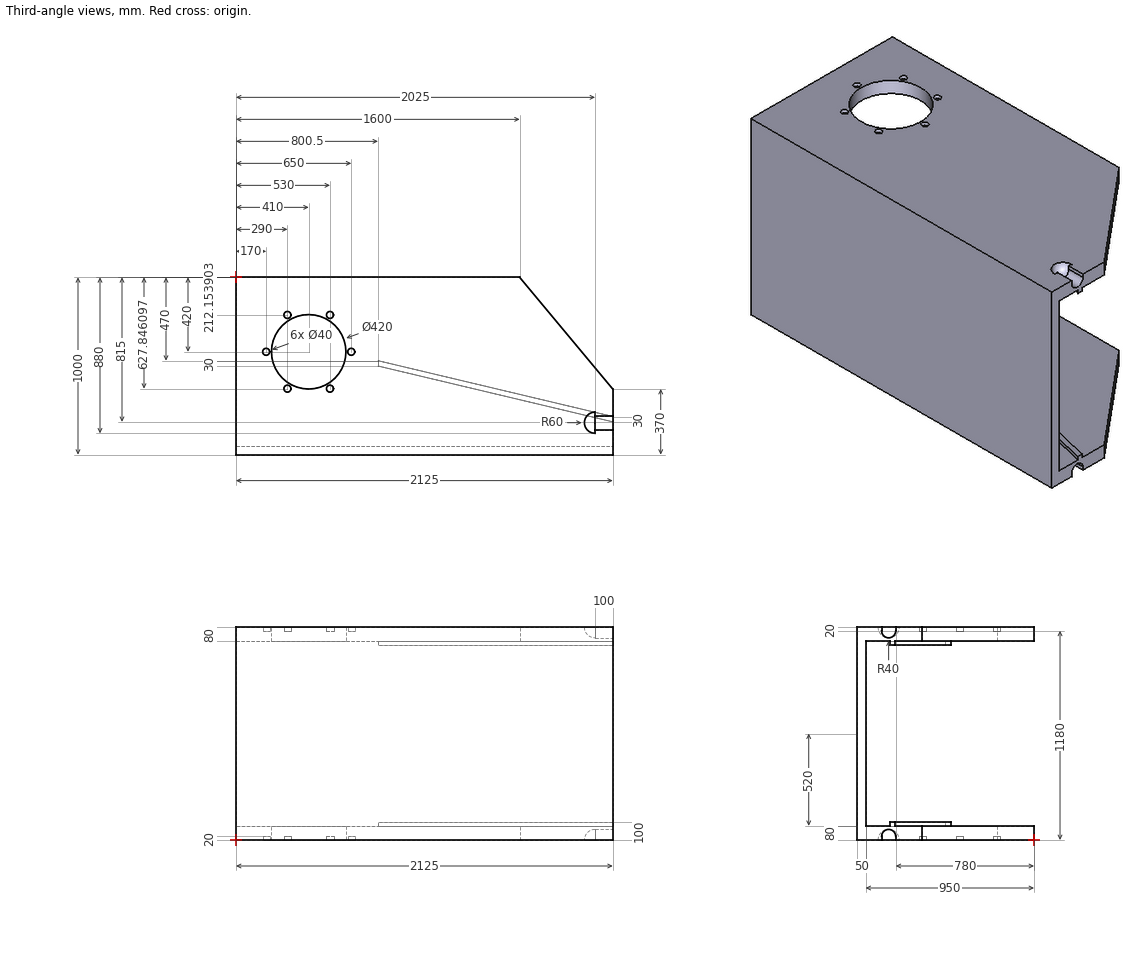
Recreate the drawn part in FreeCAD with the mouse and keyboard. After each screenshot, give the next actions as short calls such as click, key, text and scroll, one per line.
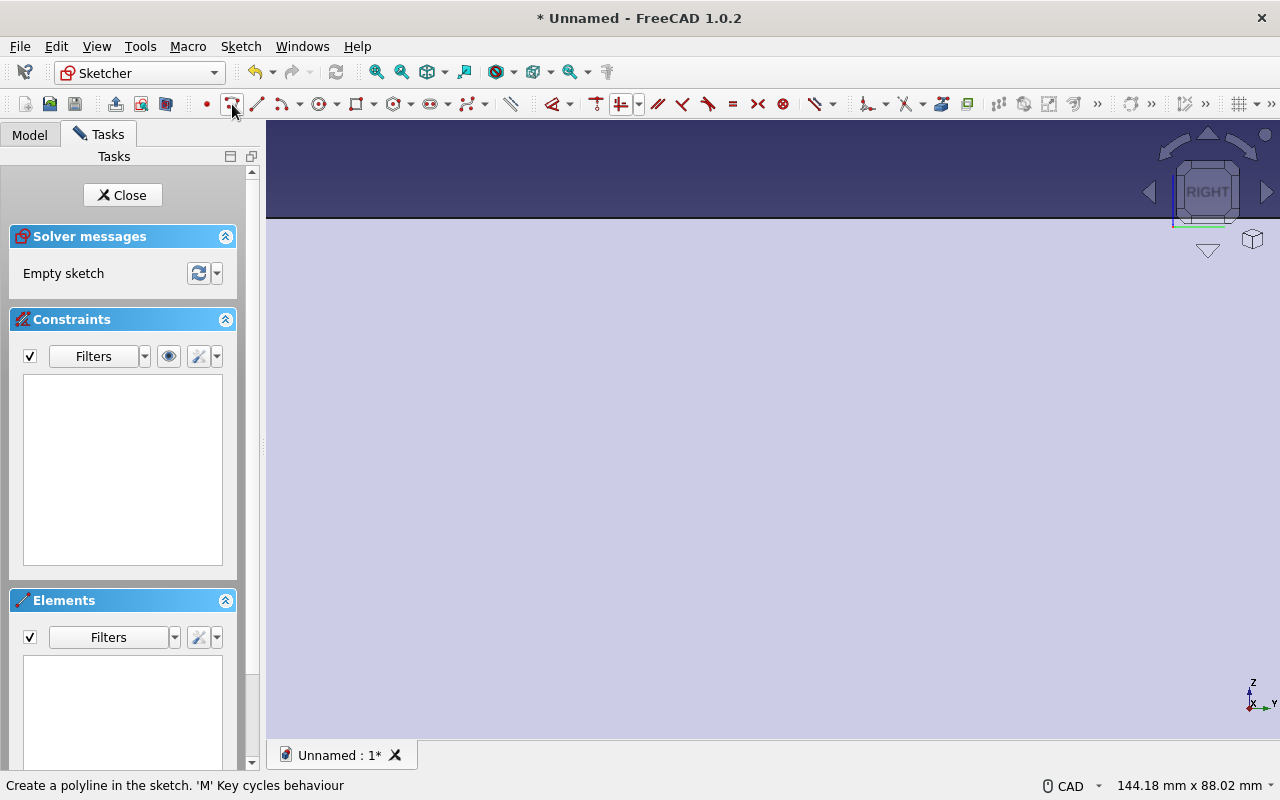
click(985, 359)
click(985, 218)
click(423, 218)
click(423, 359)
right_click(423, 359)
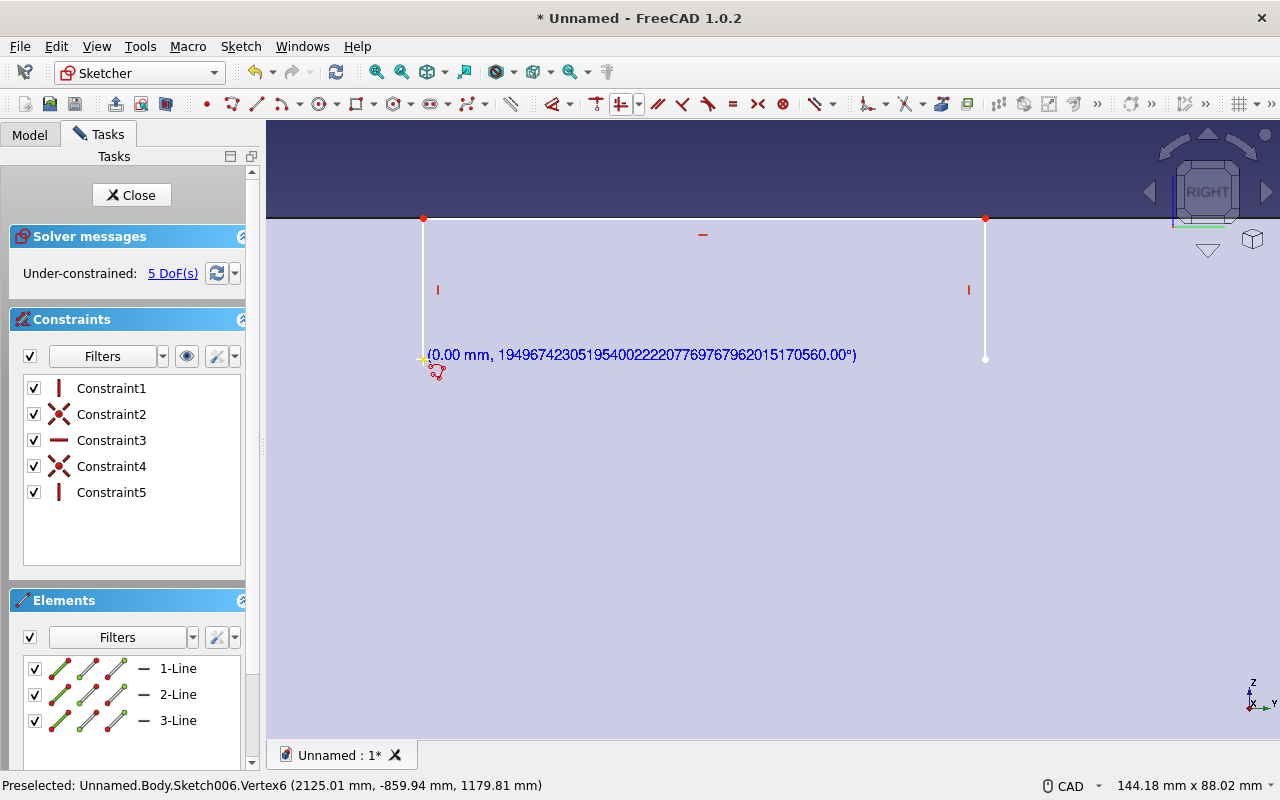
key(g)
key(3)
key(a)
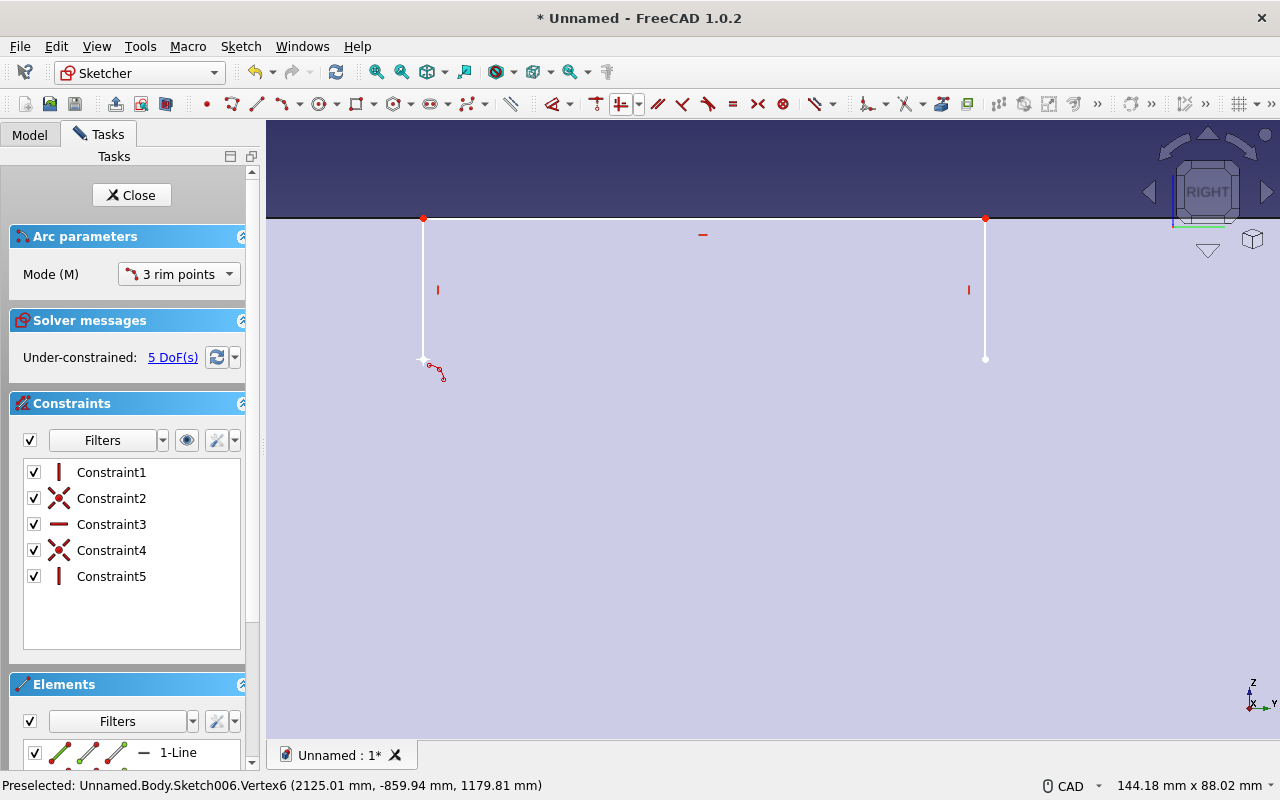
click(423, 360)
click(985, 360)
click(704, 640)
key(Escape)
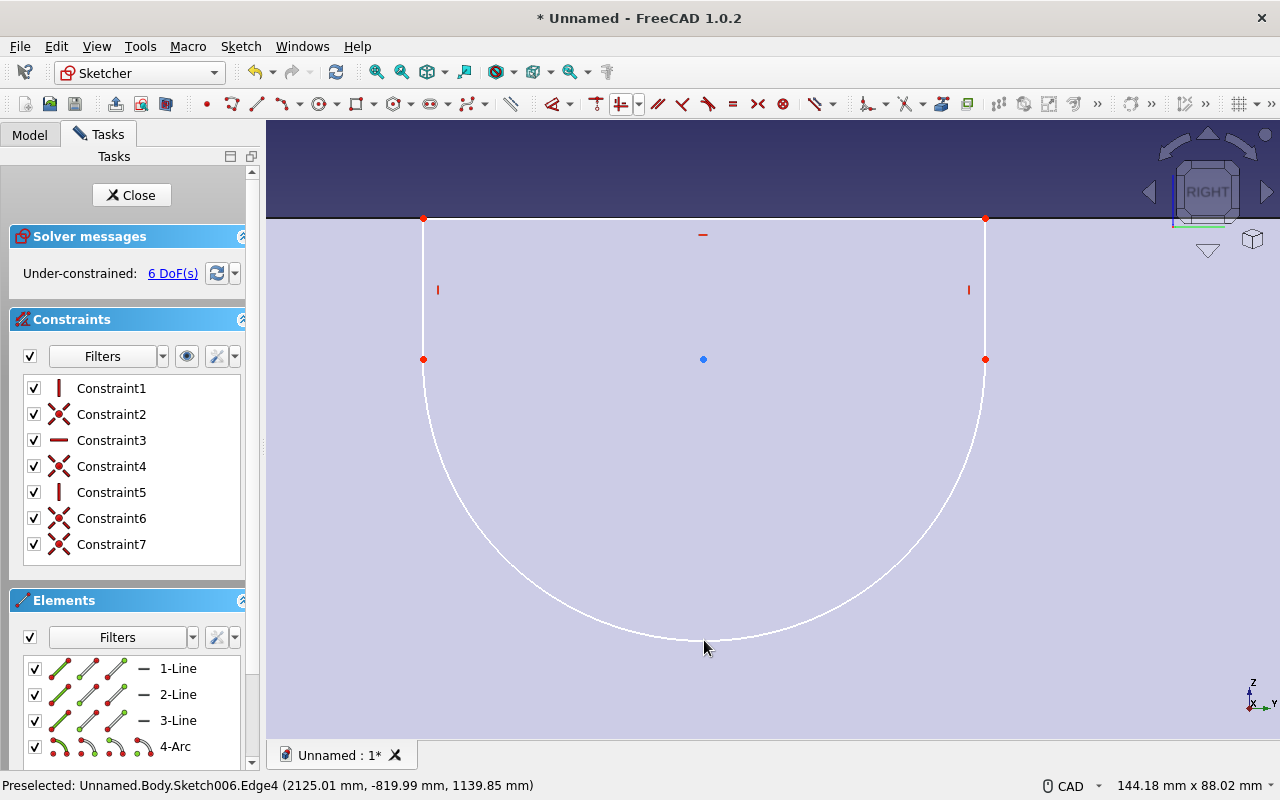
key(d)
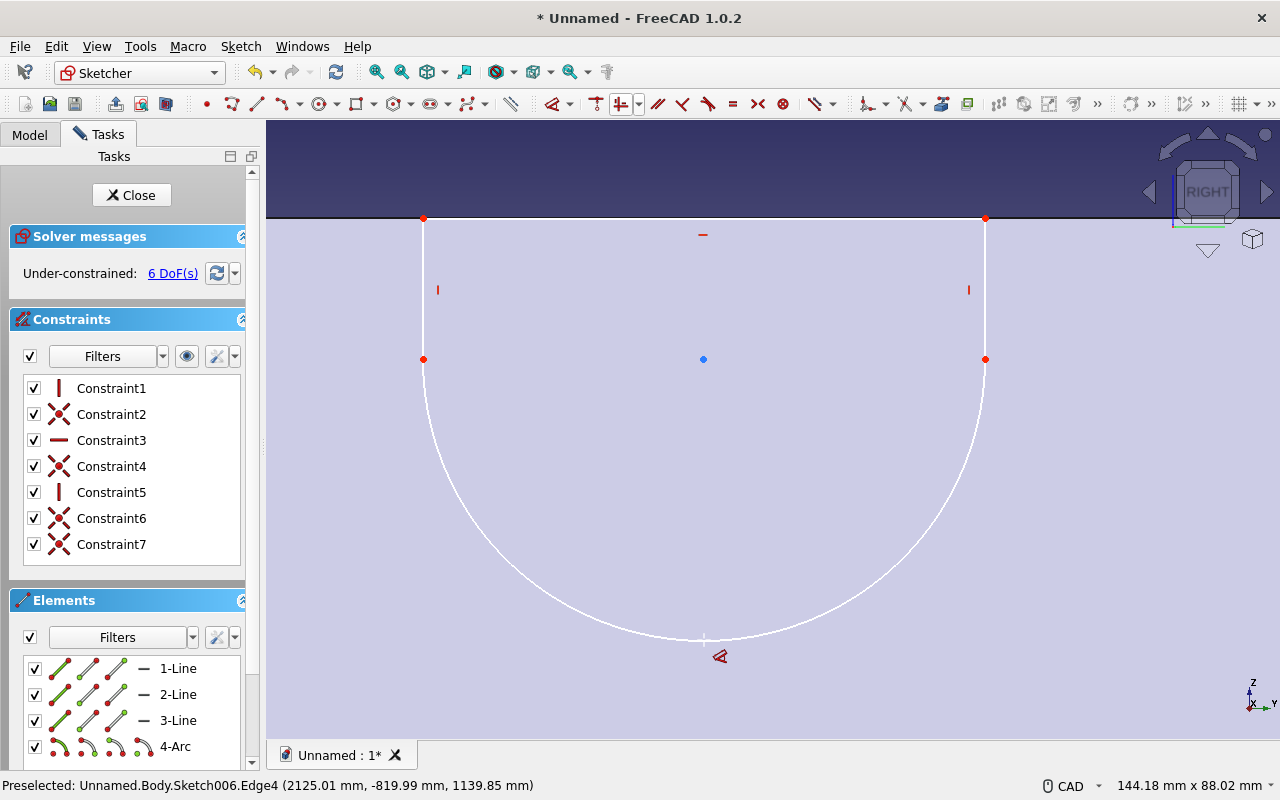
click(539, 587)
click(520, 613)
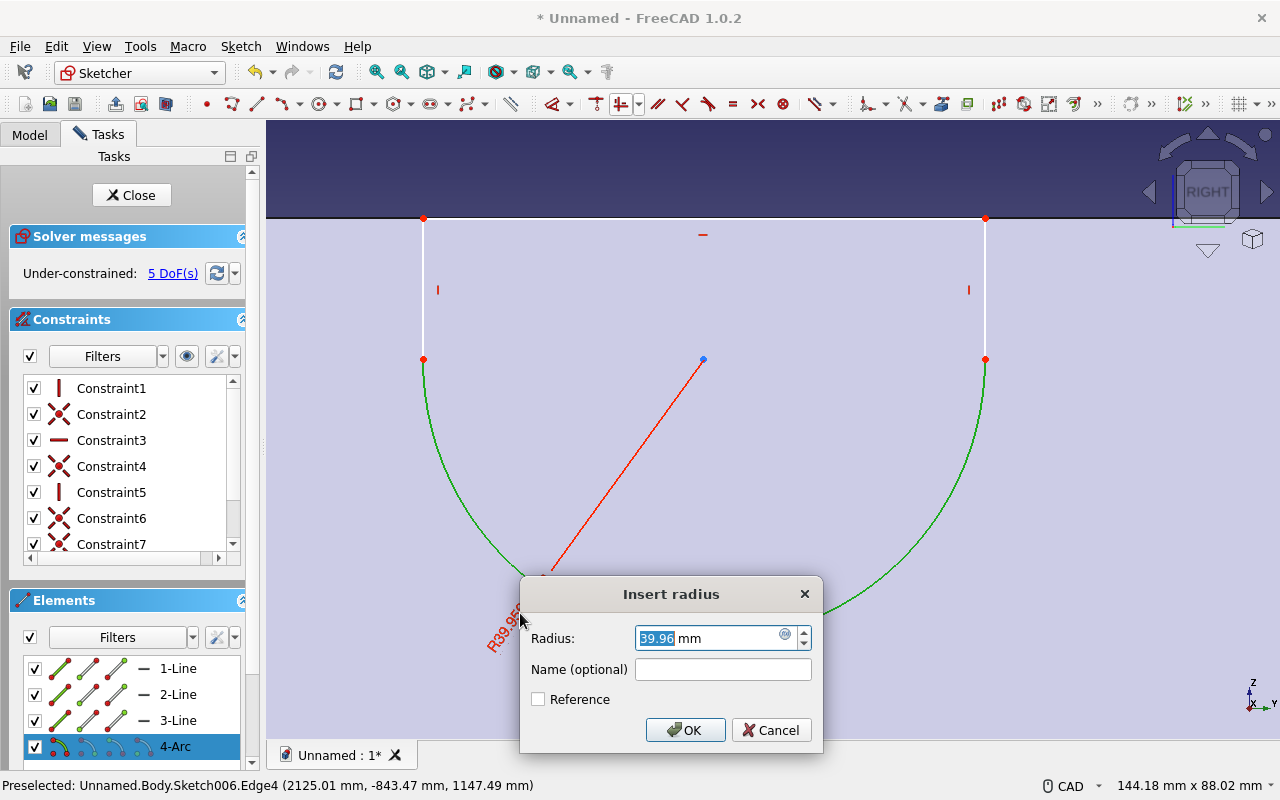
text(40)
key(Return)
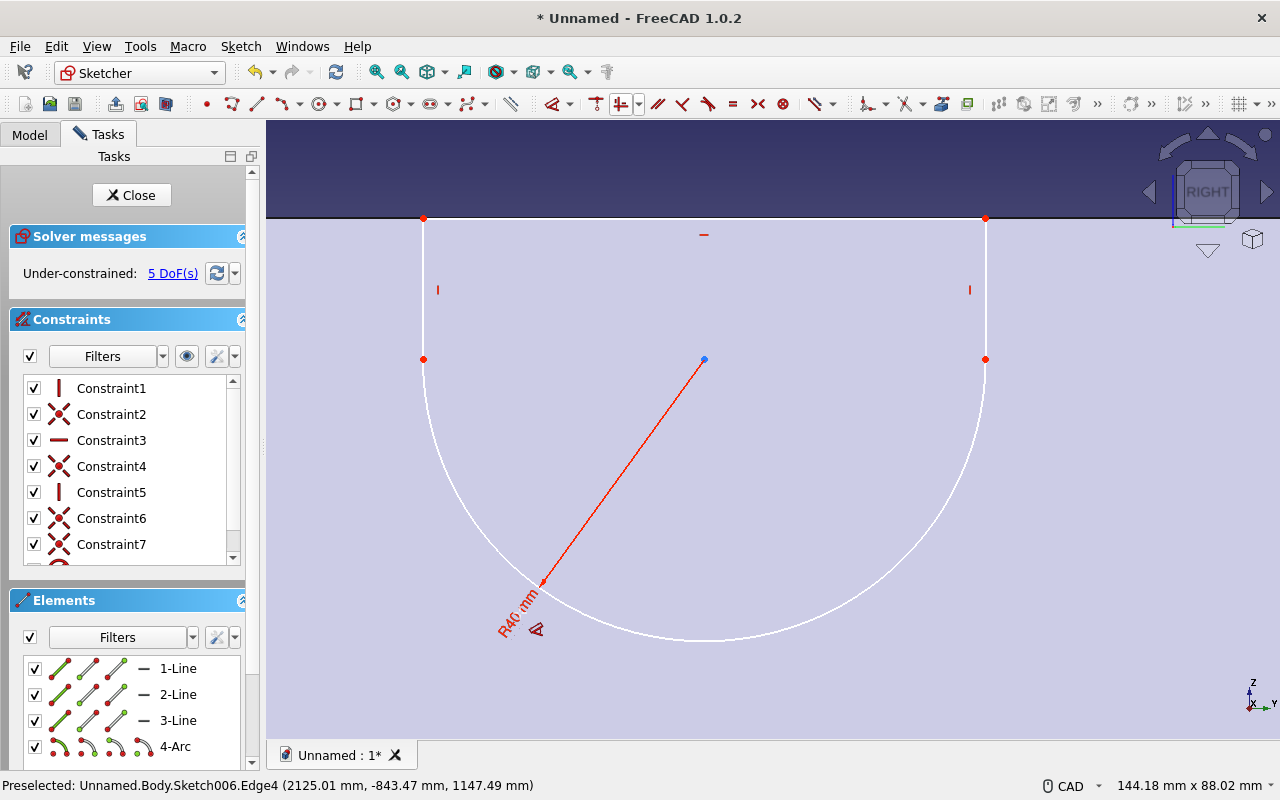
click(986, 318)
click(1020, 290)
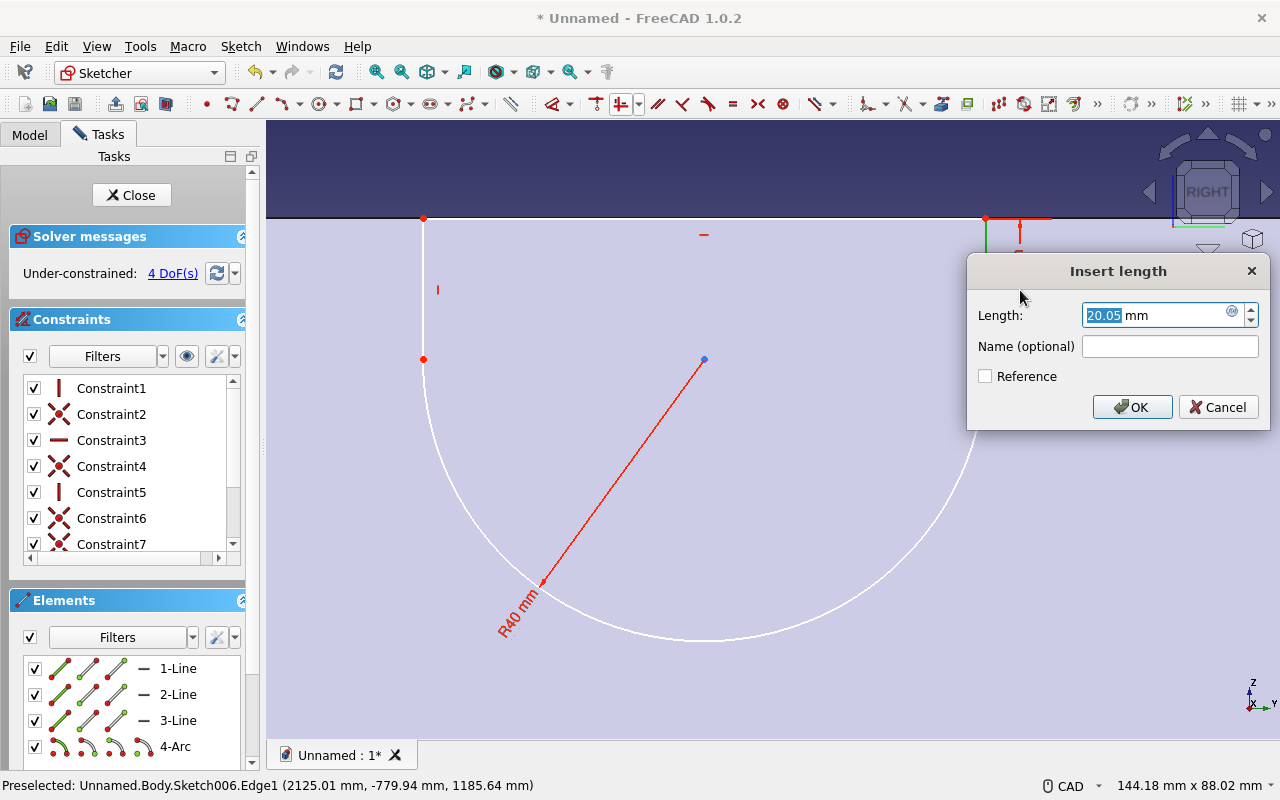
text(20)
key(Return)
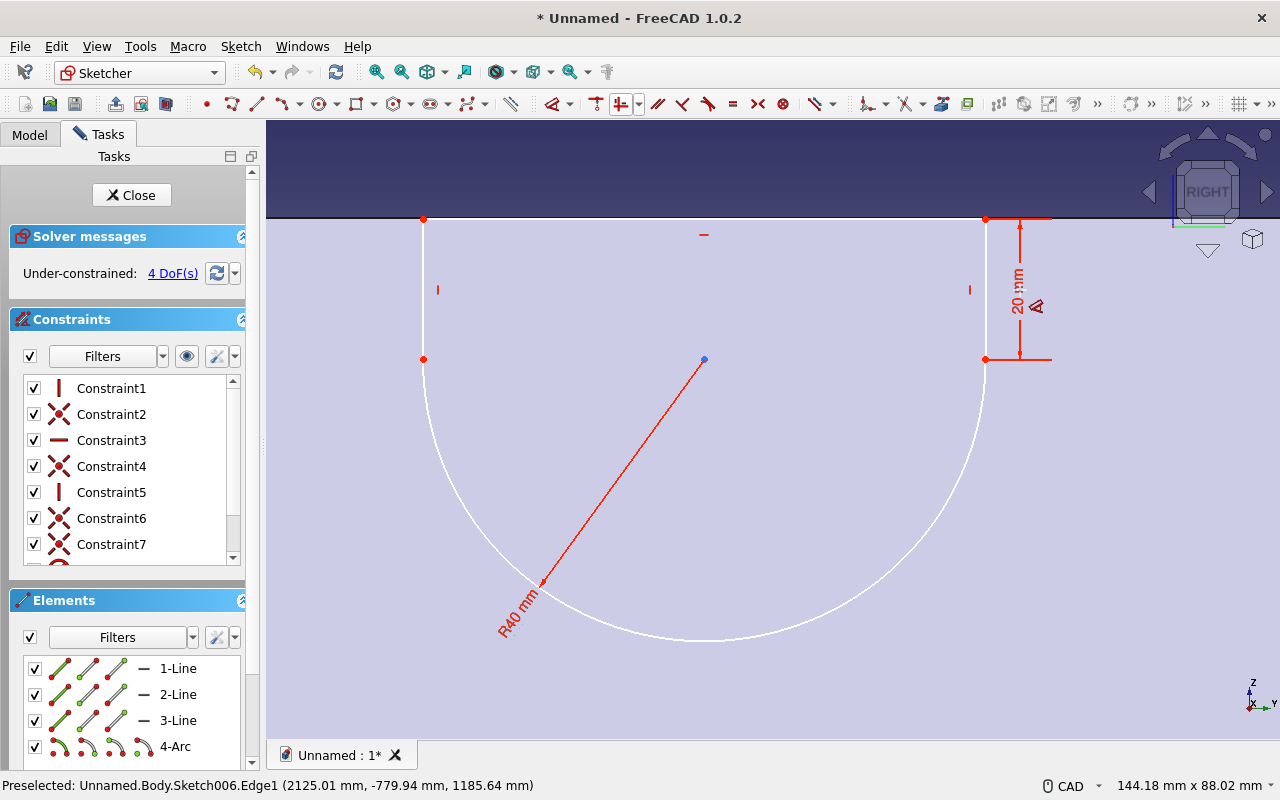
click(423, 262)
click(389, 290)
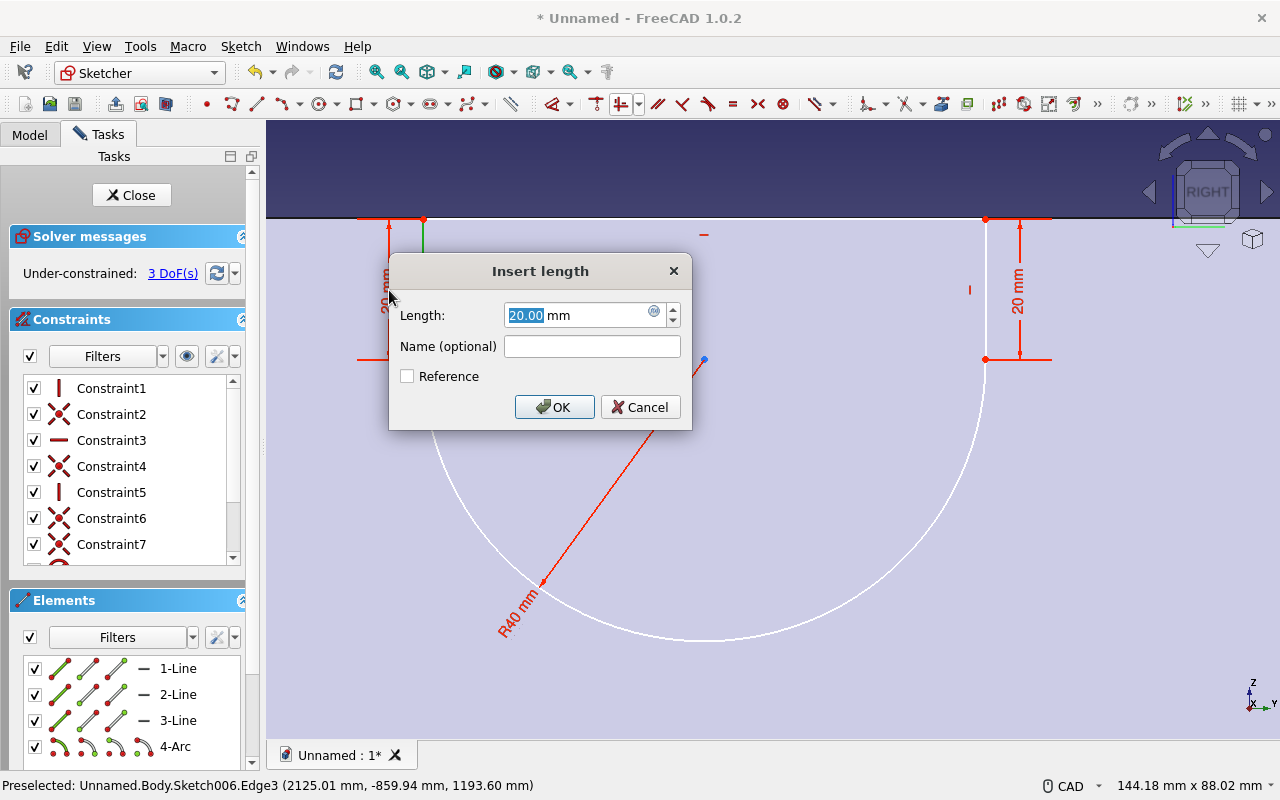
text(20)
key(Return)